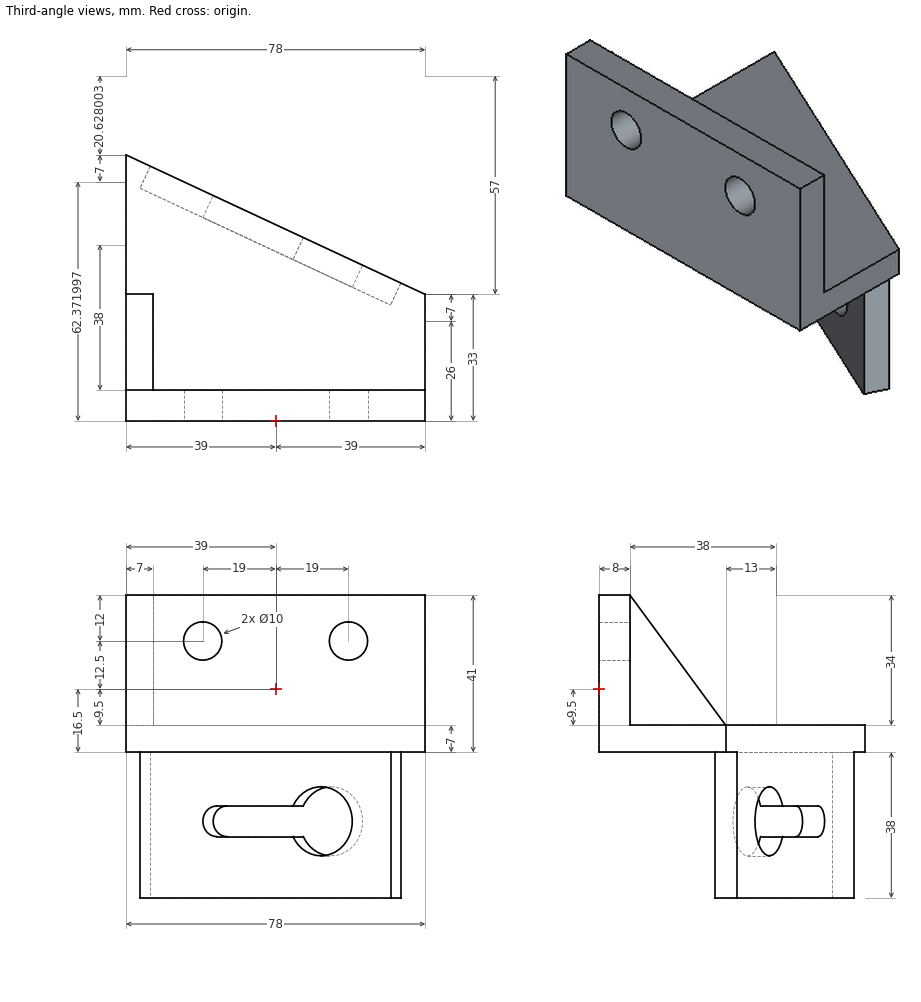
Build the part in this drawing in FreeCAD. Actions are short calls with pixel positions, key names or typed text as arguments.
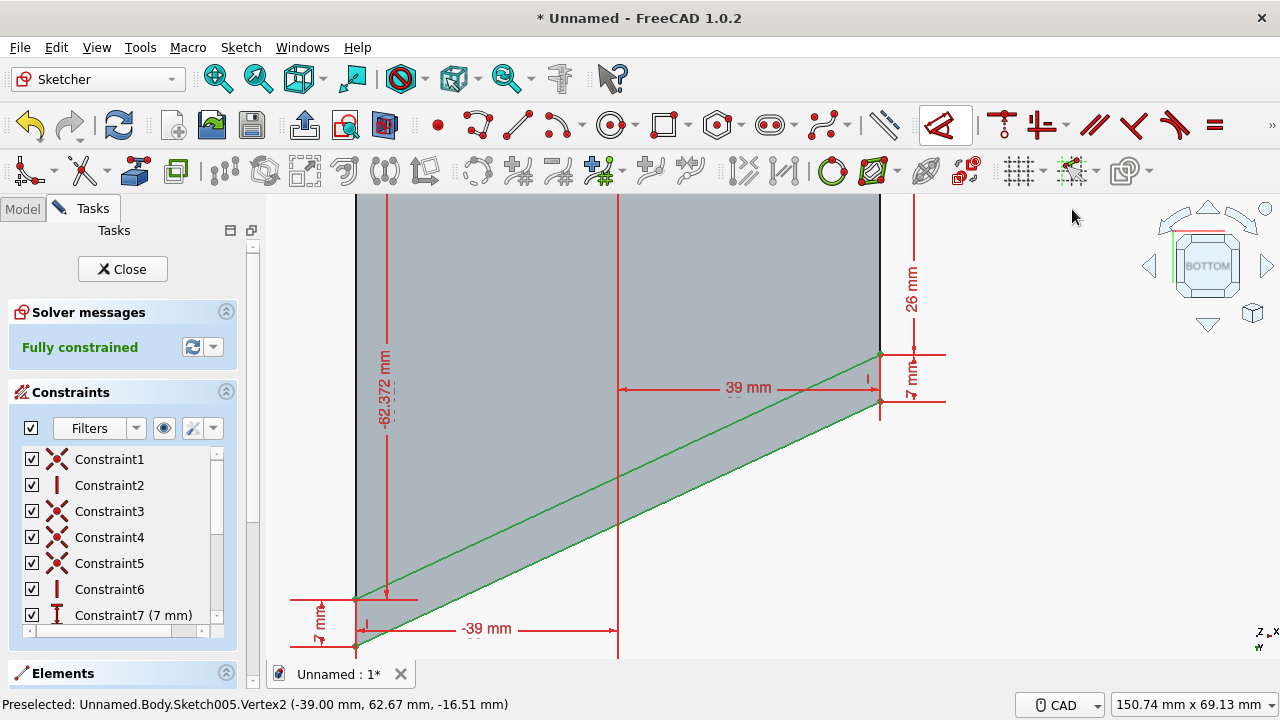
click(123, 269)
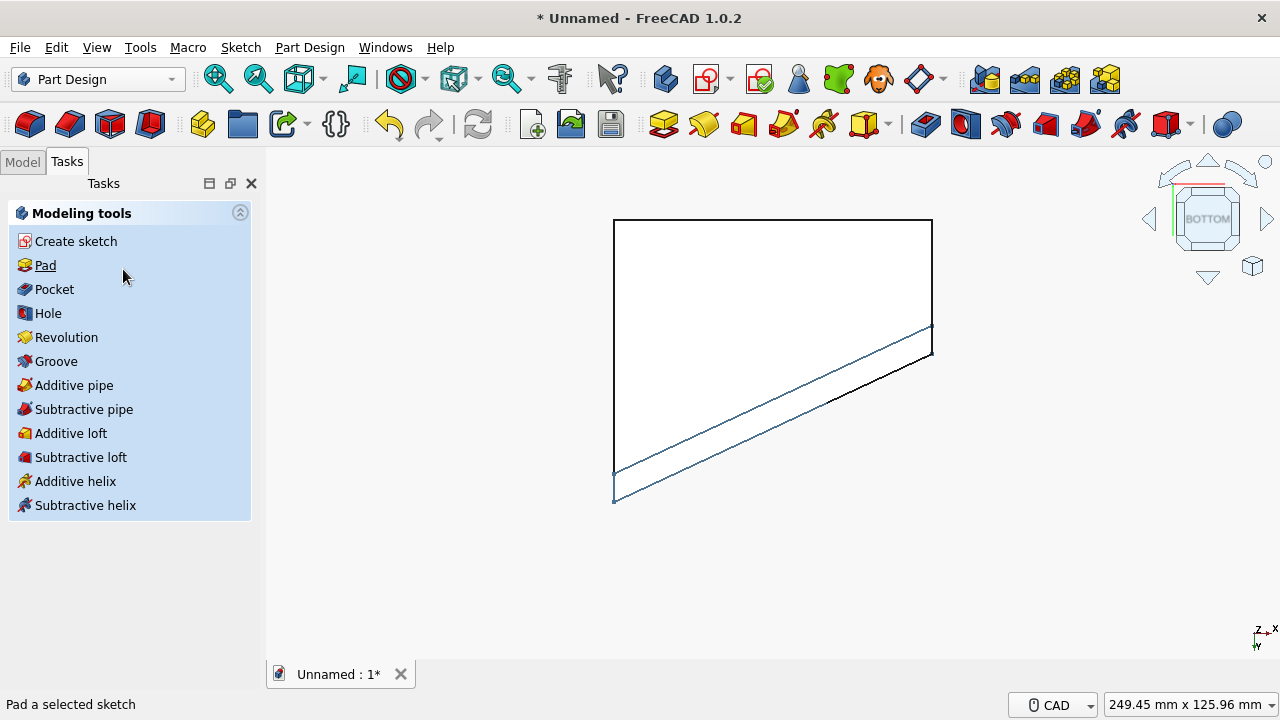
click(664, 124)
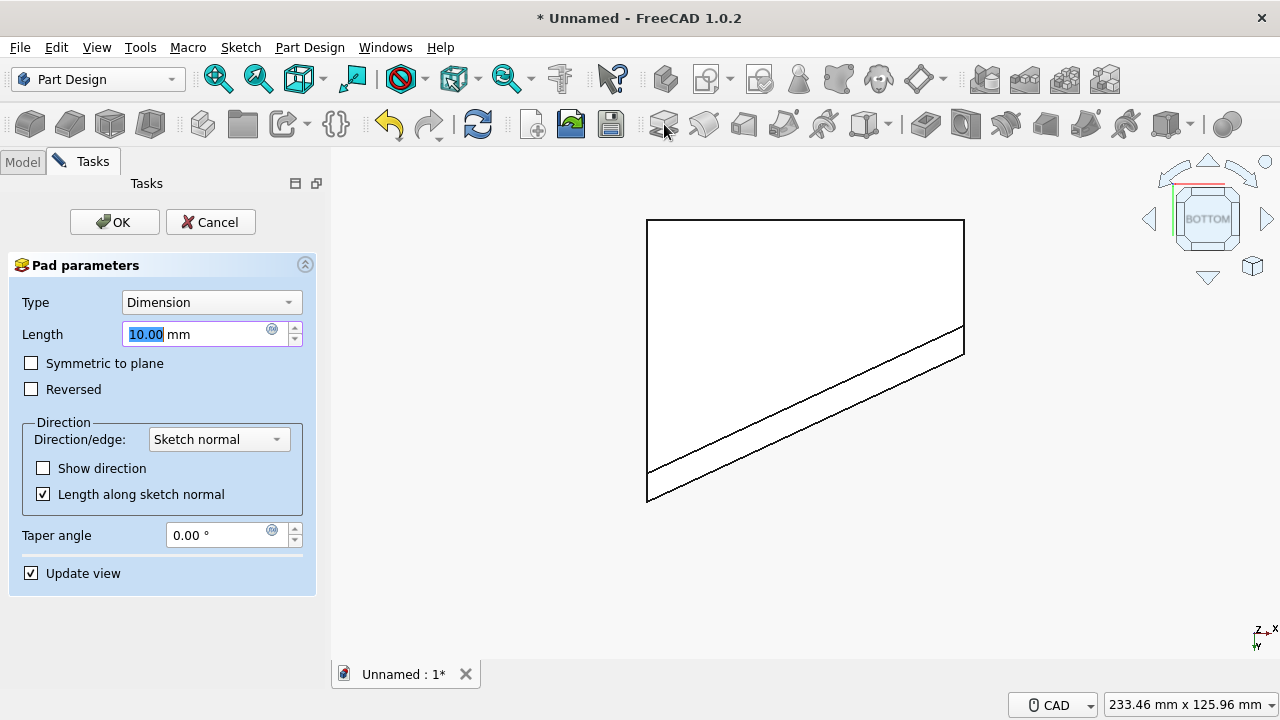
text(38)
key(Tab)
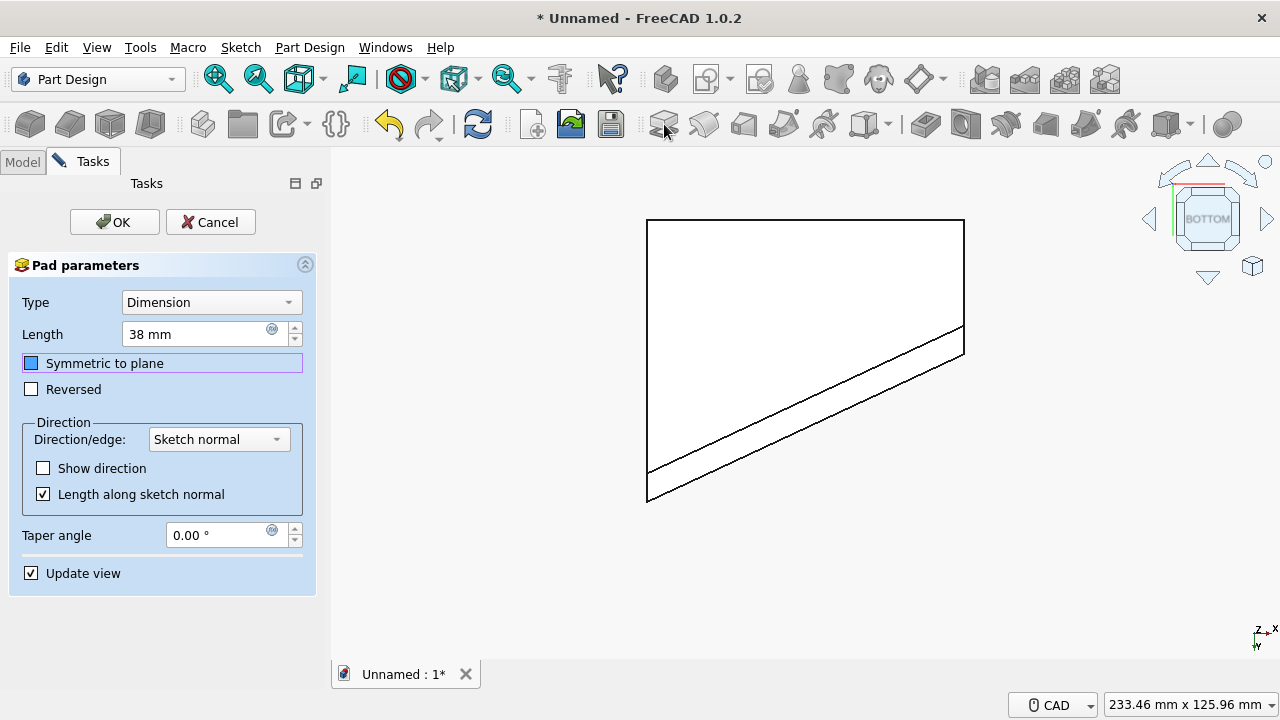
click(115, 222)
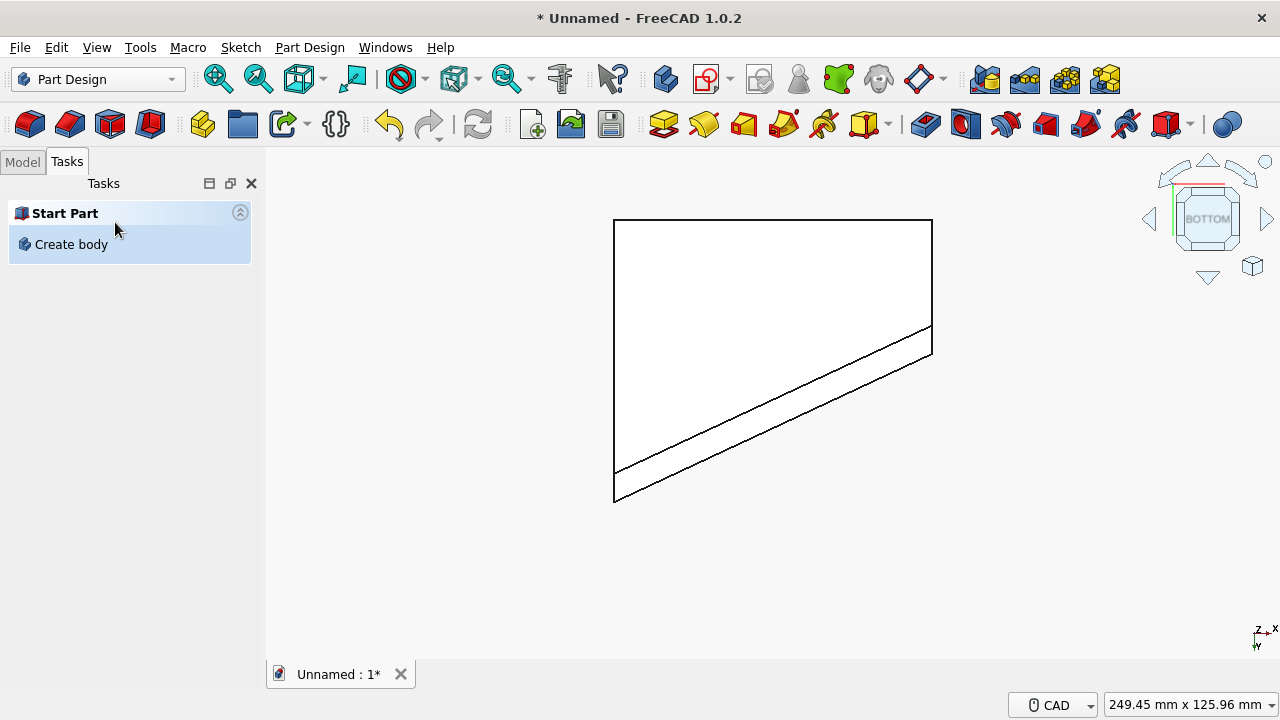
key(4)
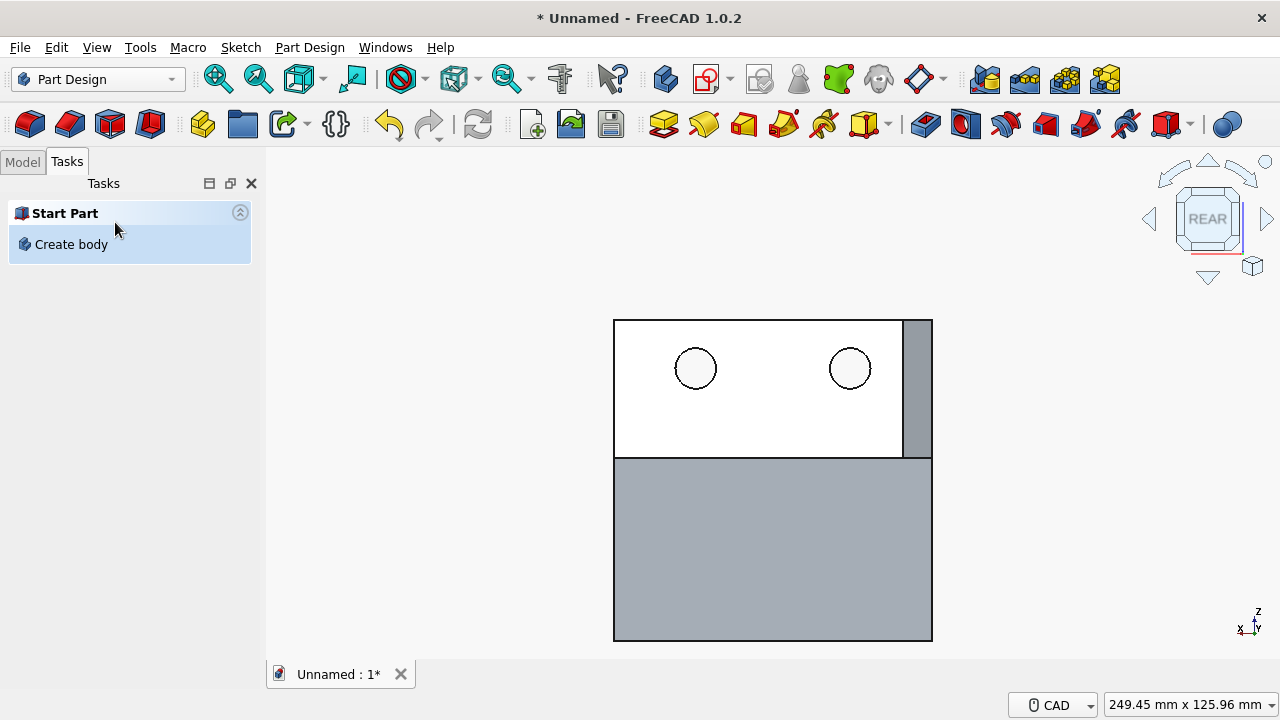
click(728, 548)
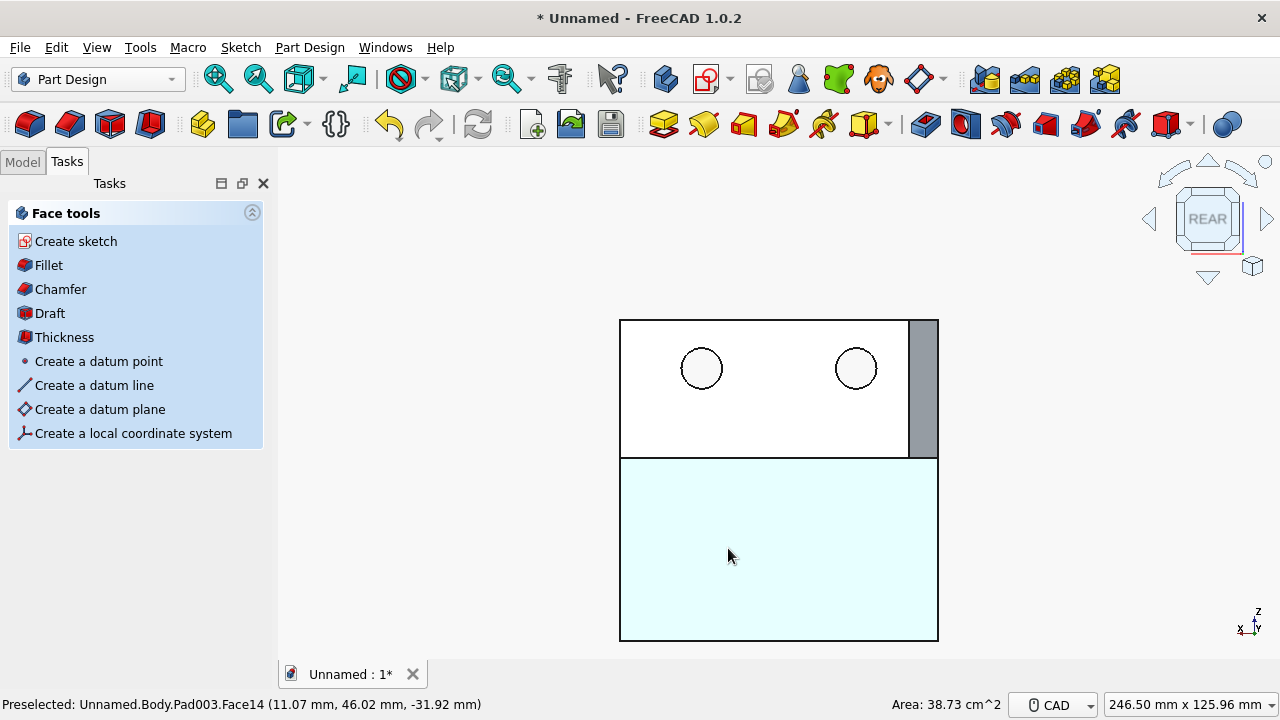
click(706, 80)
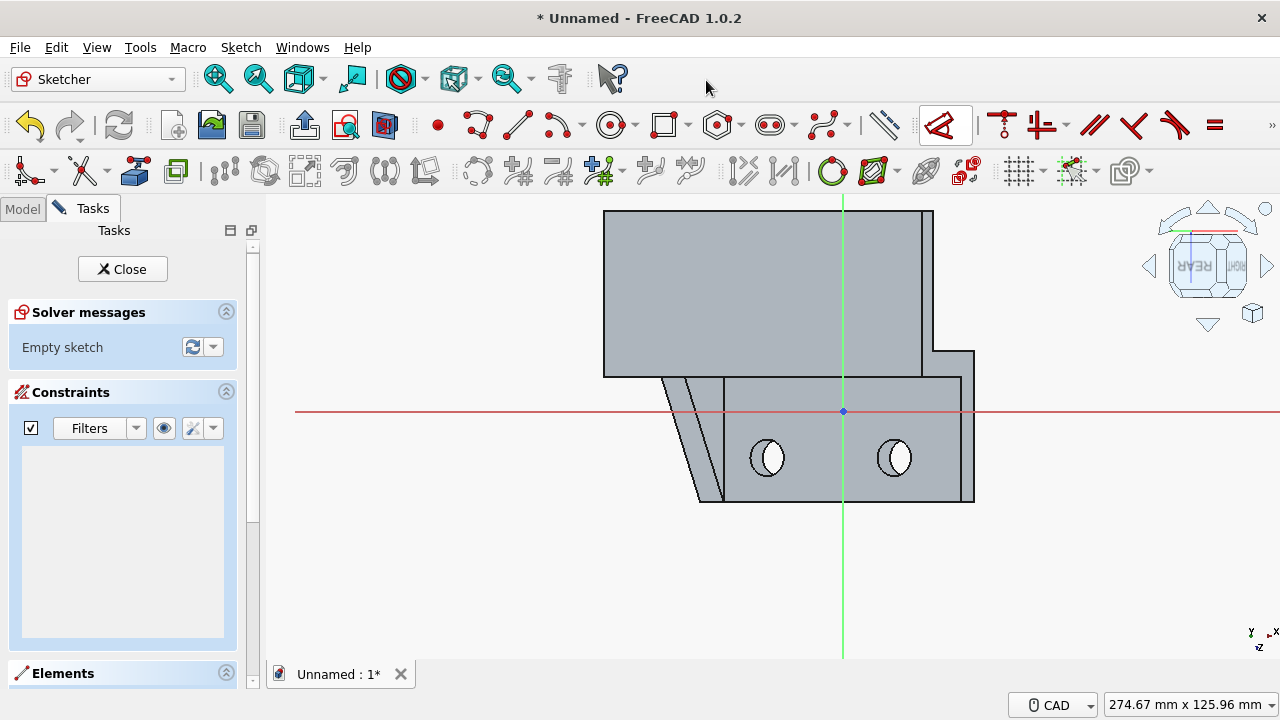
click(386, 126)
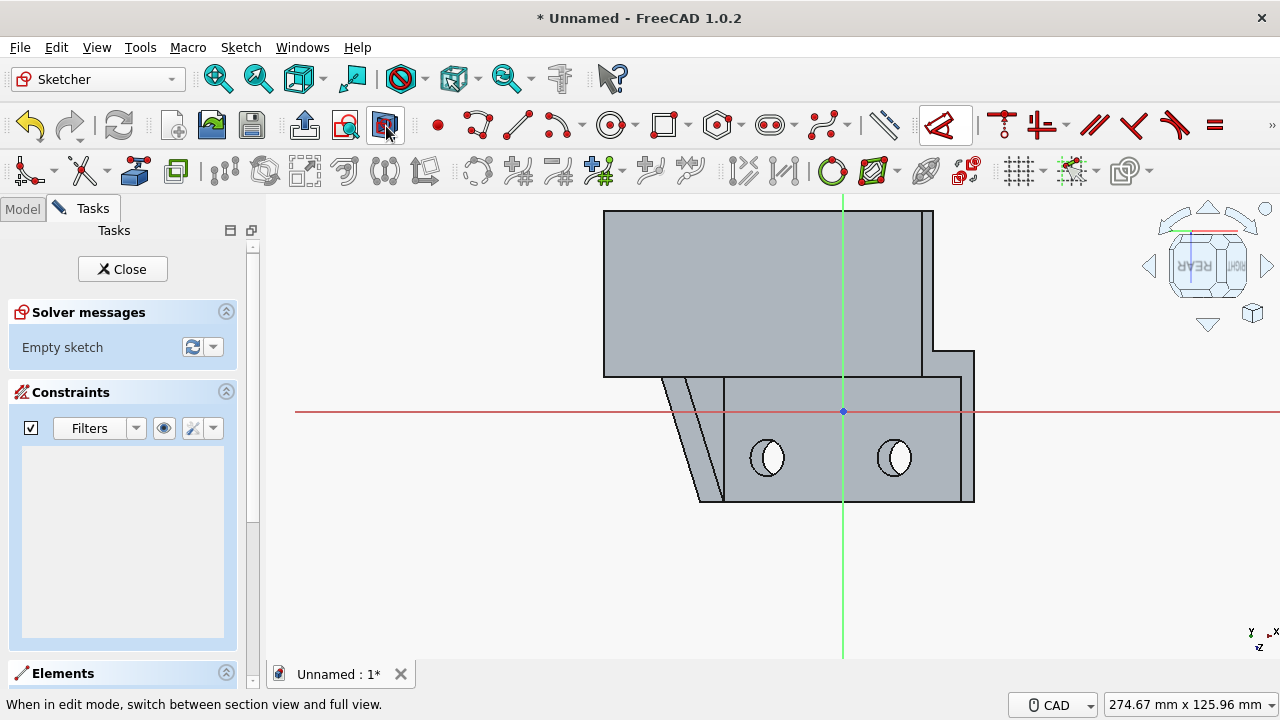
scroll(414, 631, down, 1)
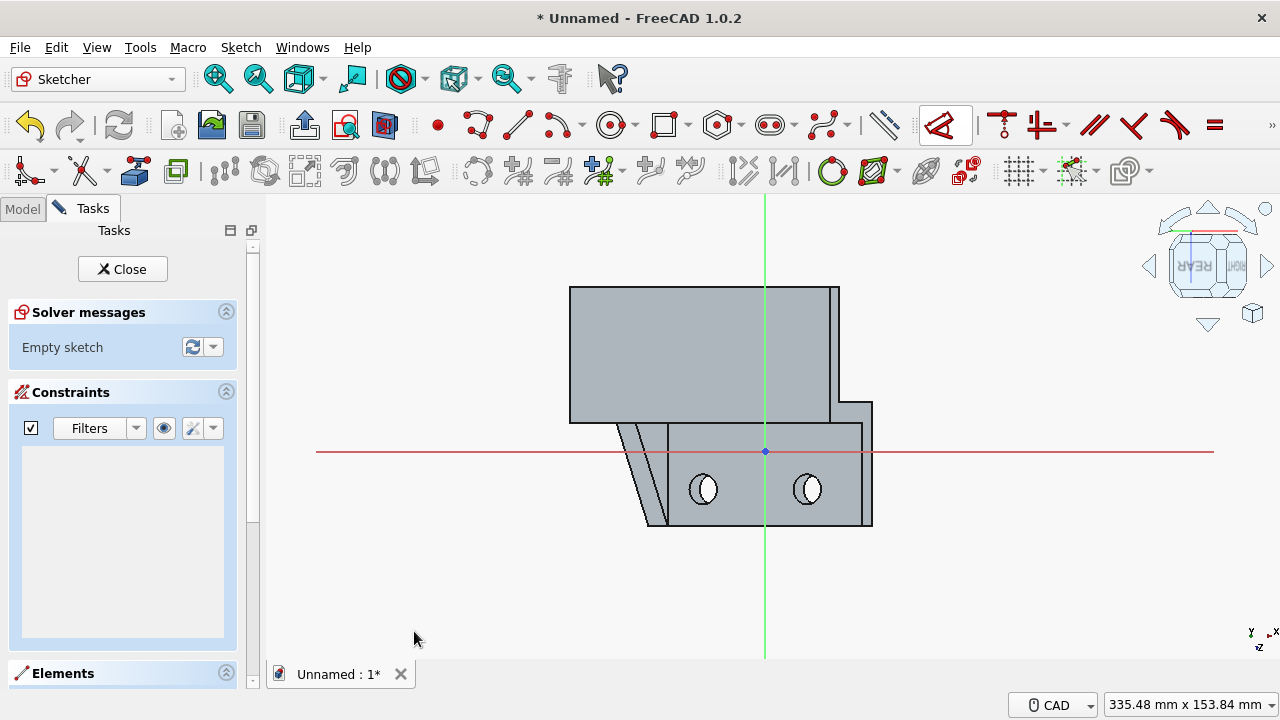
scroll(705, 300, up, 3)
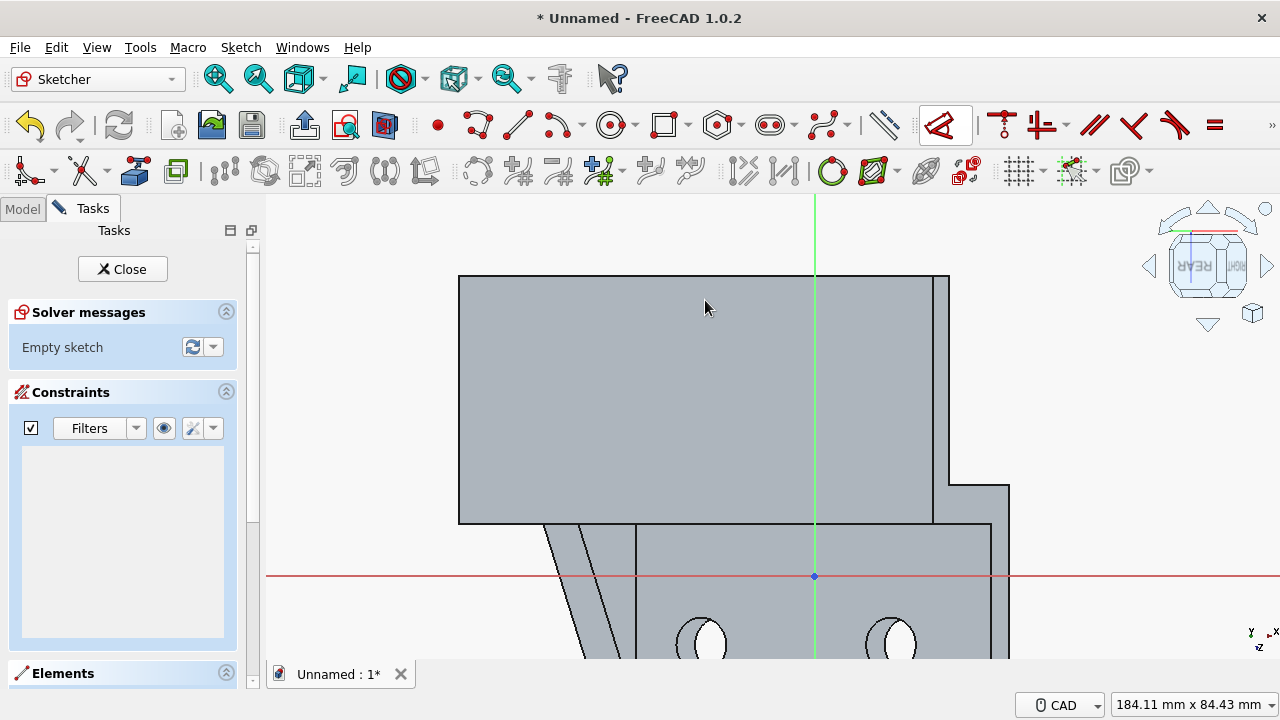
click(664, 126)